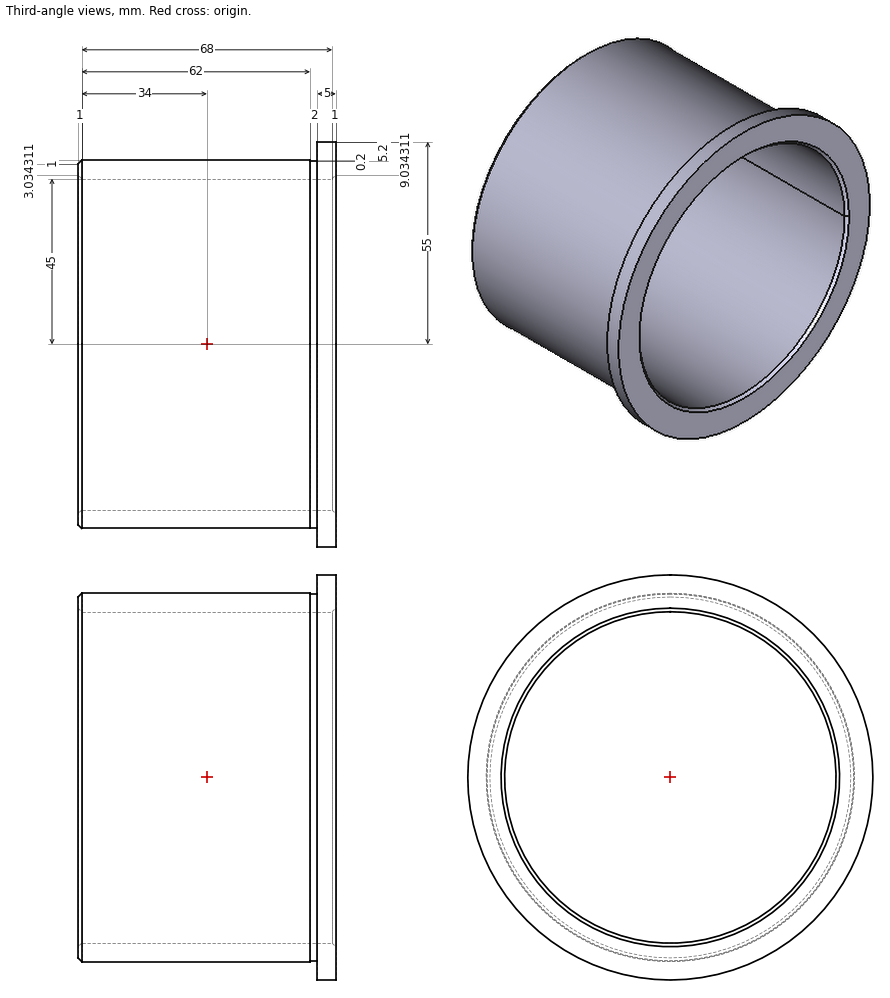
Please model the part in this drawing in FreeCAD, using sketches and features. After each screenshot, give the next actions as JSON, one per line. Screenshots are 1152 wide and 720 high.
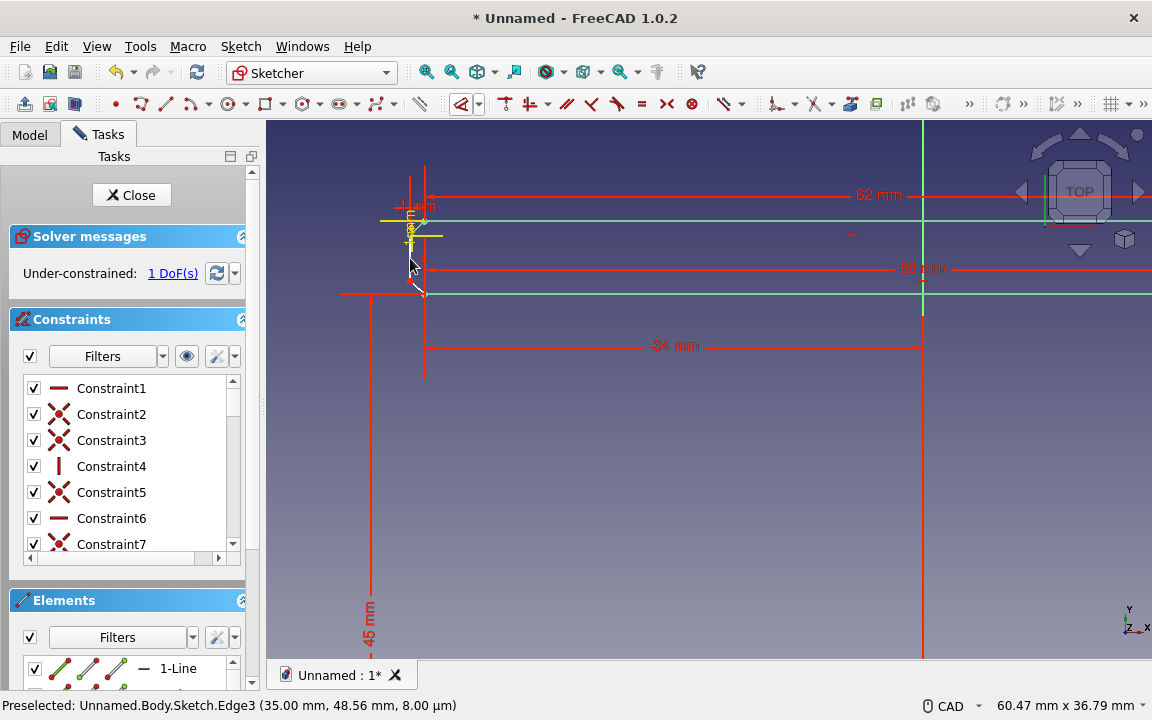
{"action": "left_click", "coordinate": [410, 259]}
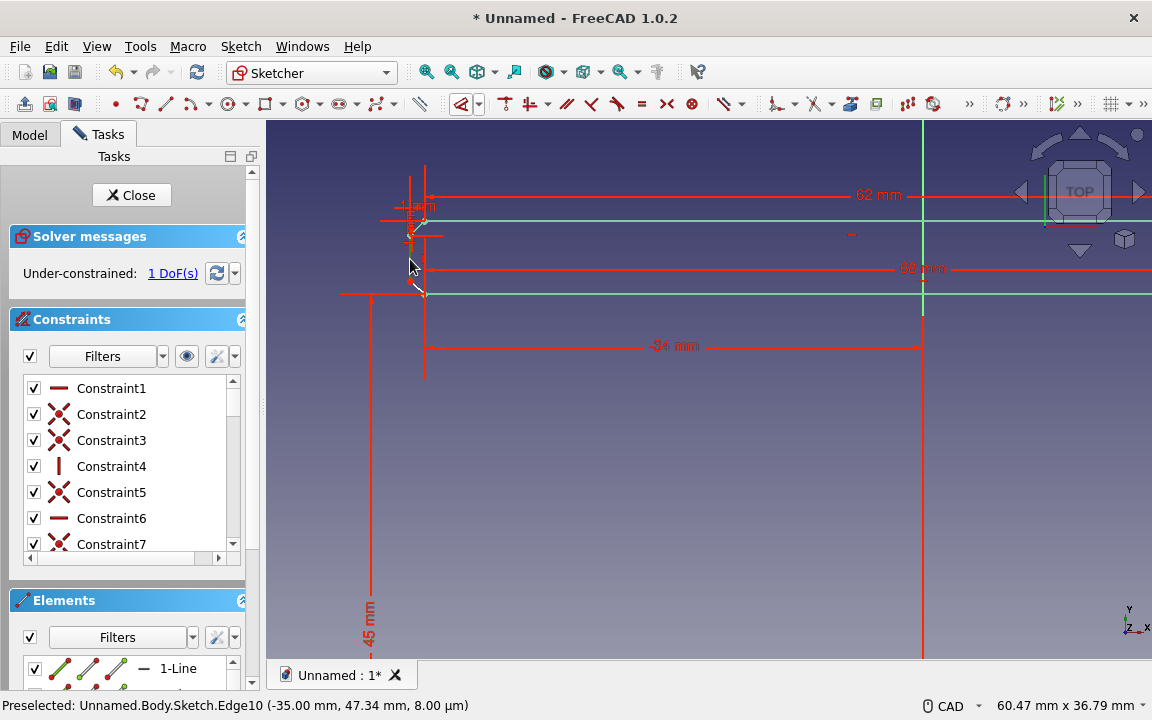
{"action": "key", "text": "i"}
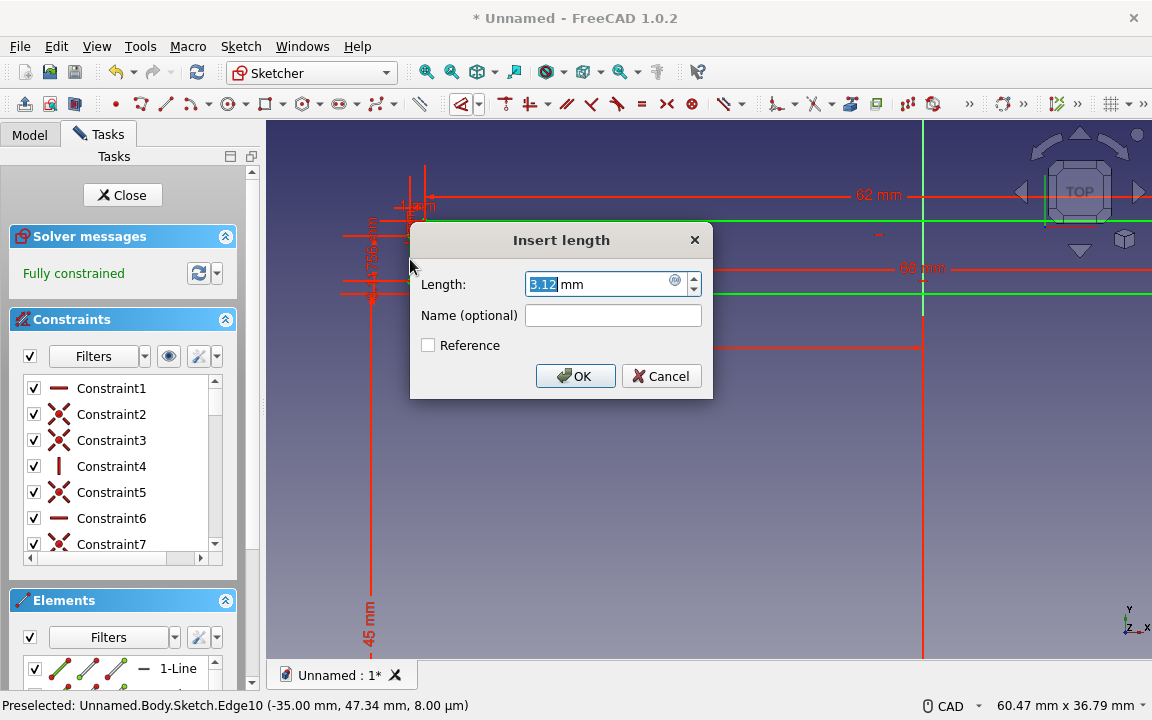
{"action": "type", "text": "3.034311"}
{"action": "key", "text": "Return"}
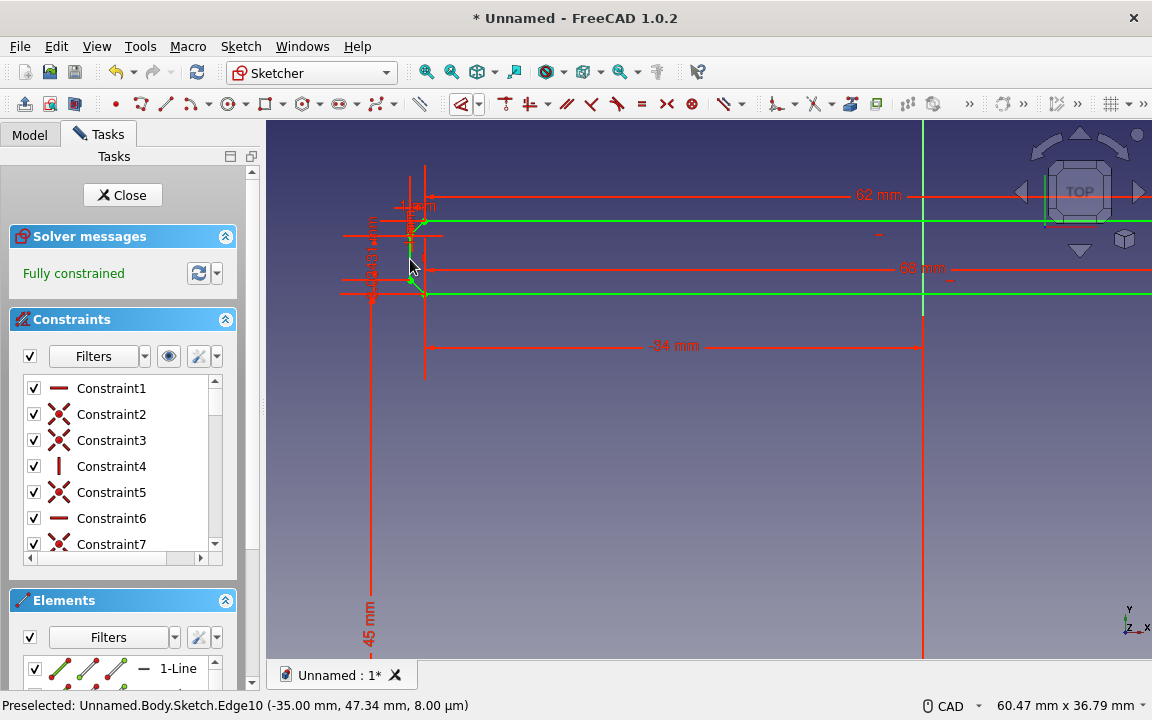
{"action": "left_click", "coordinate": [123, 195]}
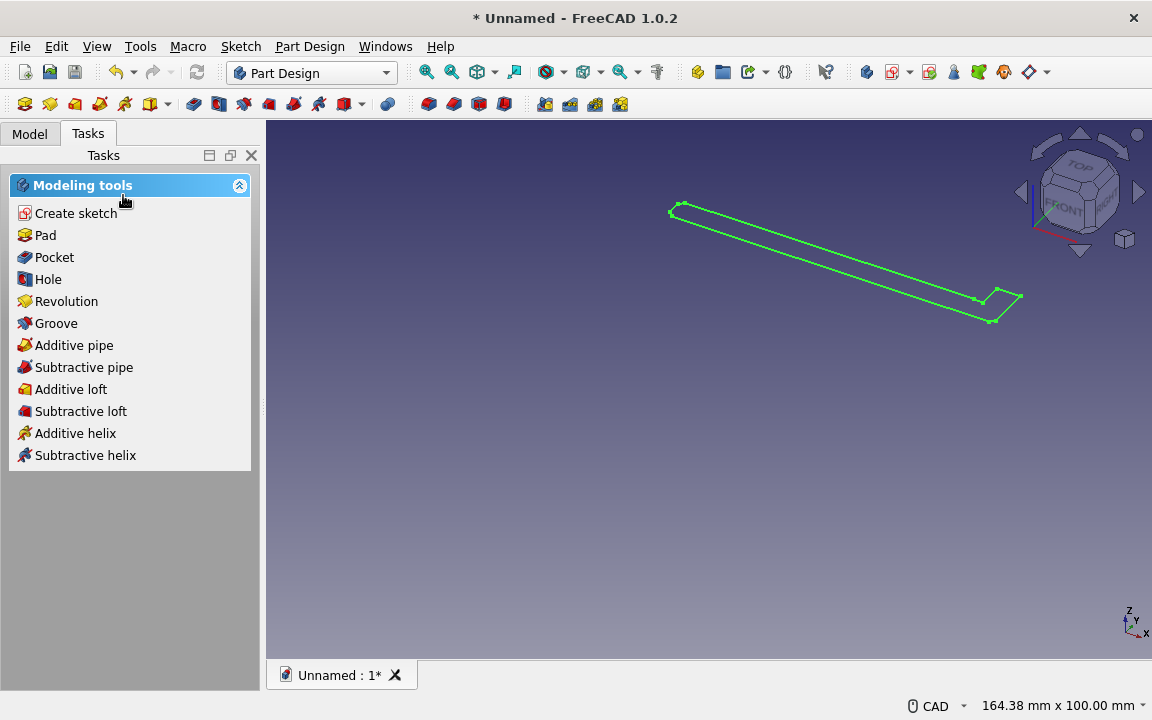
{"action": "left_click", "coordinate": [50, 104]}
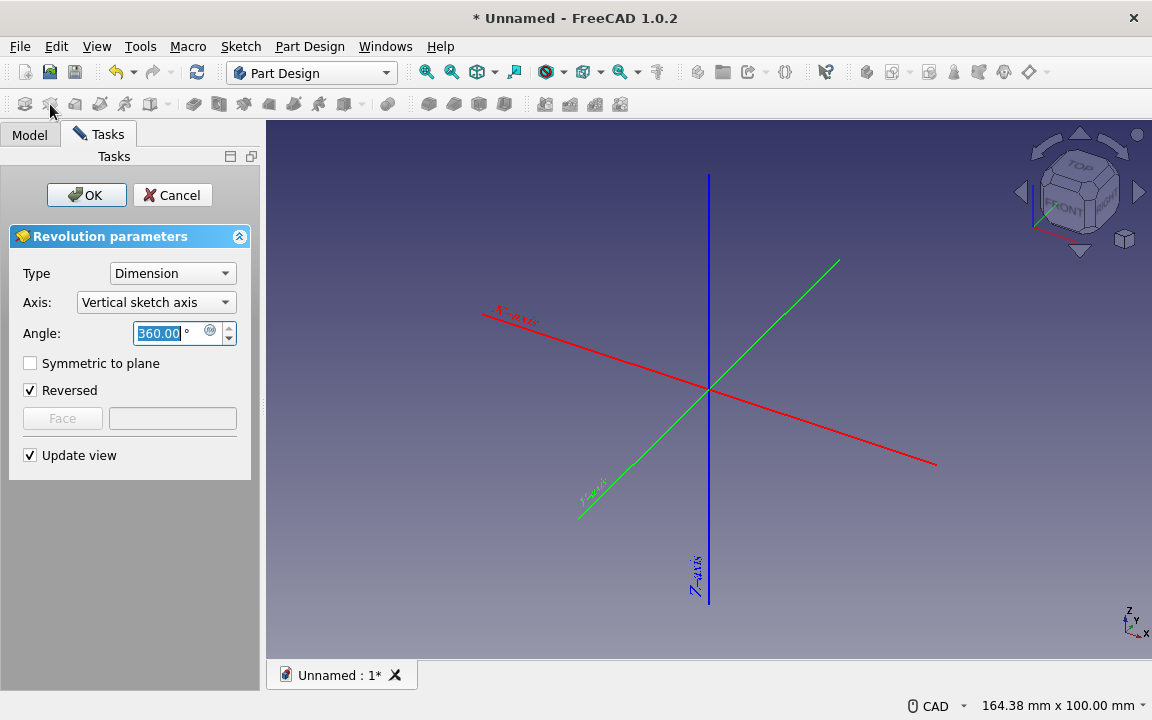
{"action": "left_click", "coordinate": [157, 302]}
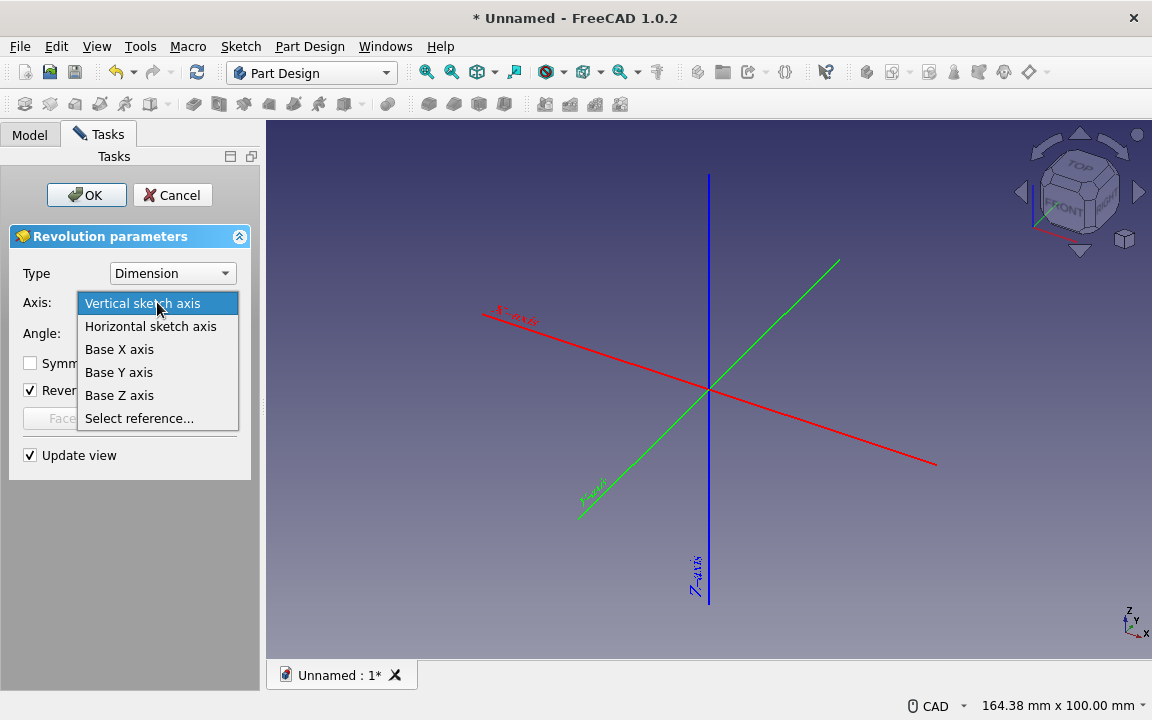
{"action": "left_click", "coordinate": [156, 326]}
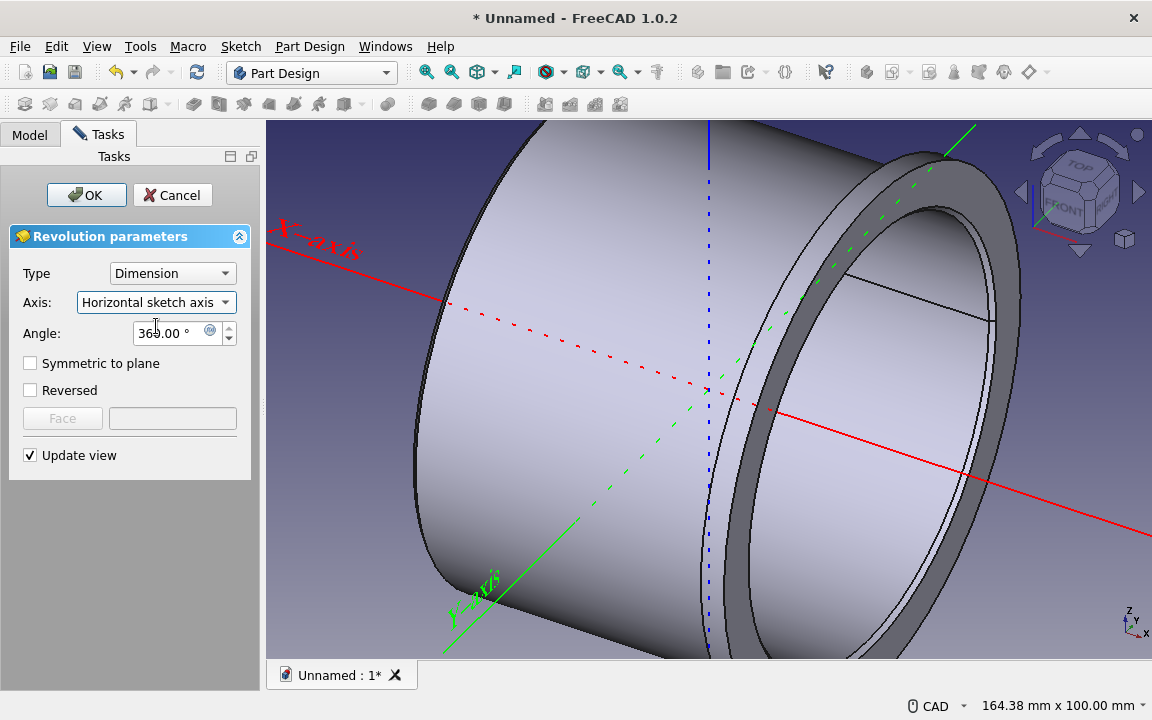
{"action": "left_click", "coordinate": [87, 195]}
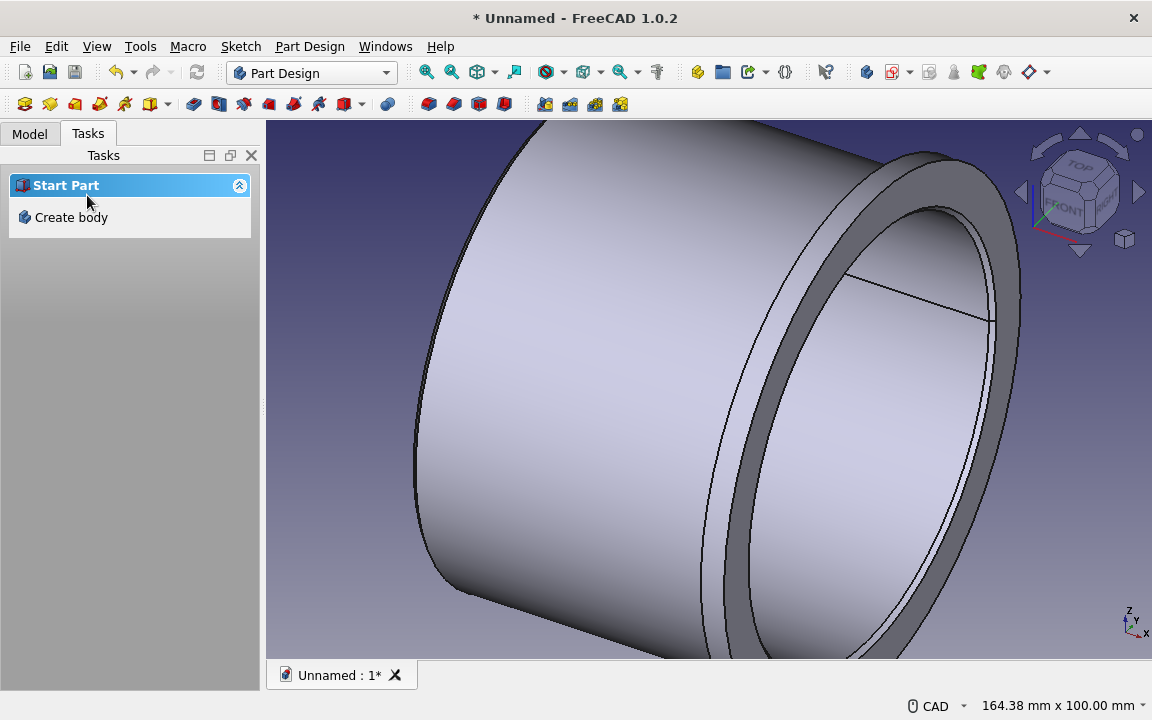
{"action": "key", "text": "0"}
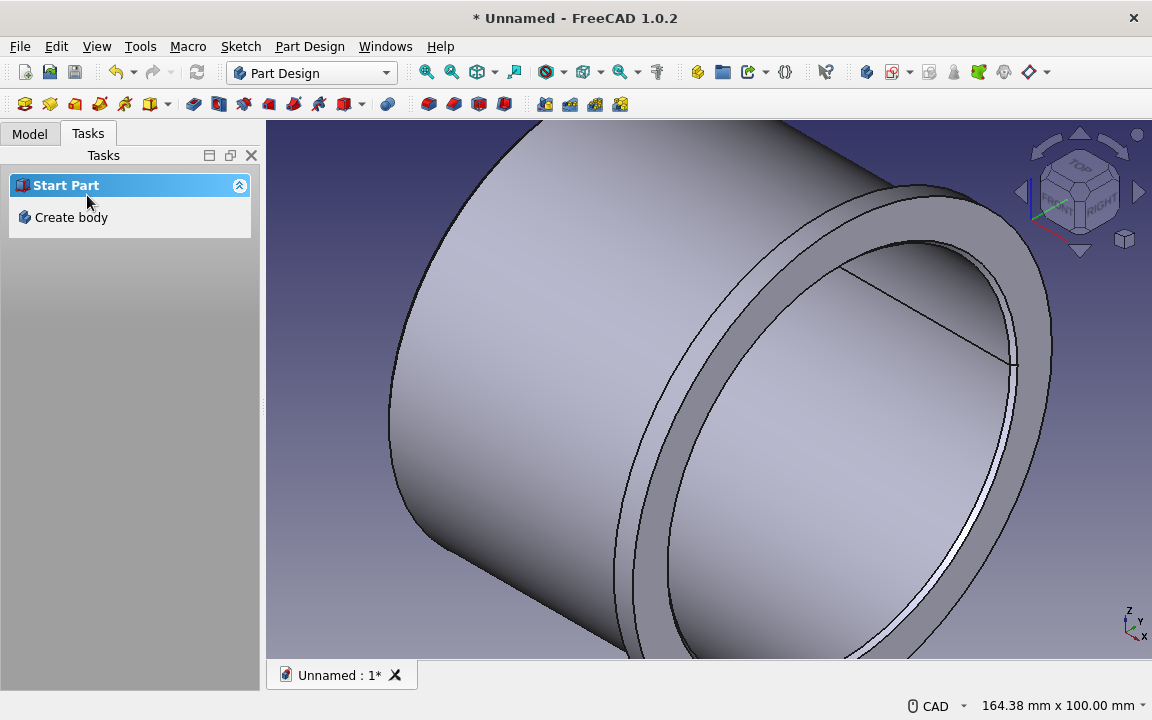
{"action": "key", "text": "v f"}